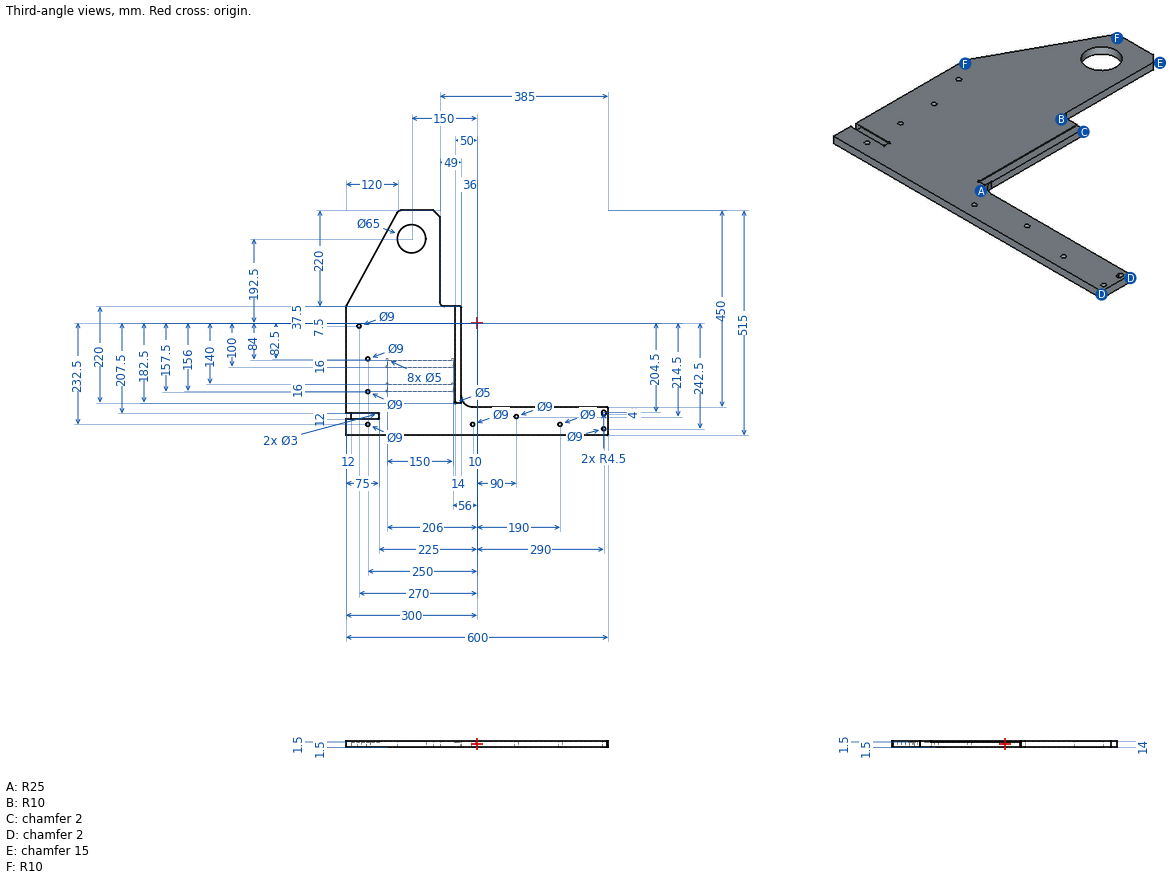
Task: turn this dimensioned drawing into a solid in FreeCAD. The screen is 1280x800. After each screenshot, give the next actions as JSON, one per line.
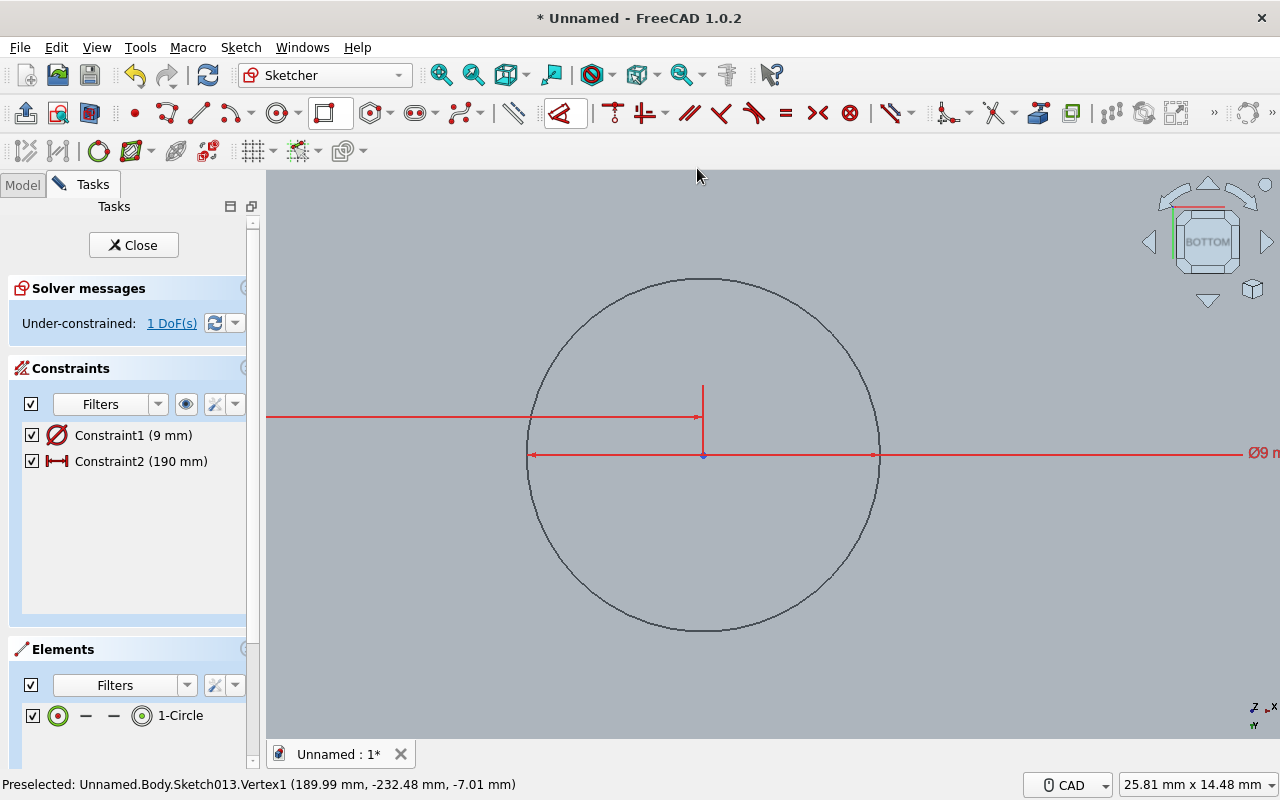
{"action": "left_click", "coordinate": [703, 455]}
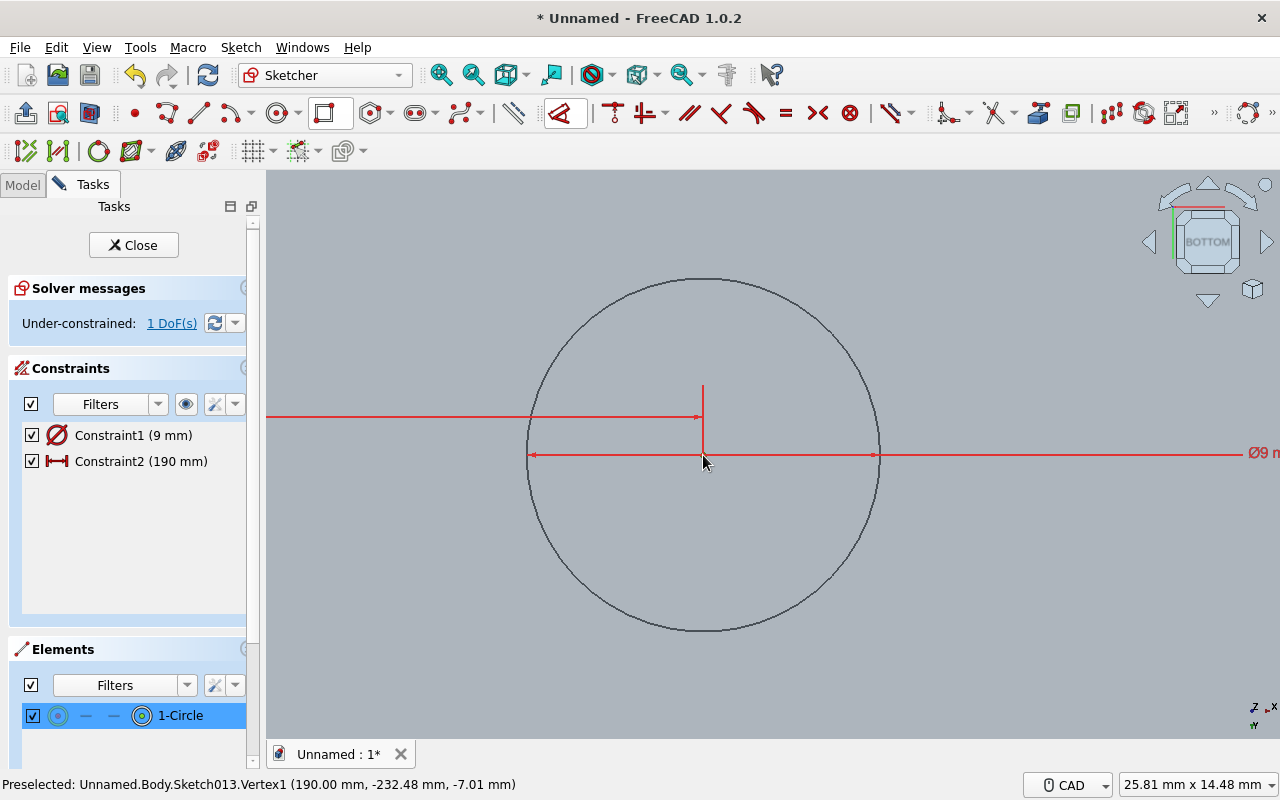
{"action": "left_click", "coordinate": [582, 114]}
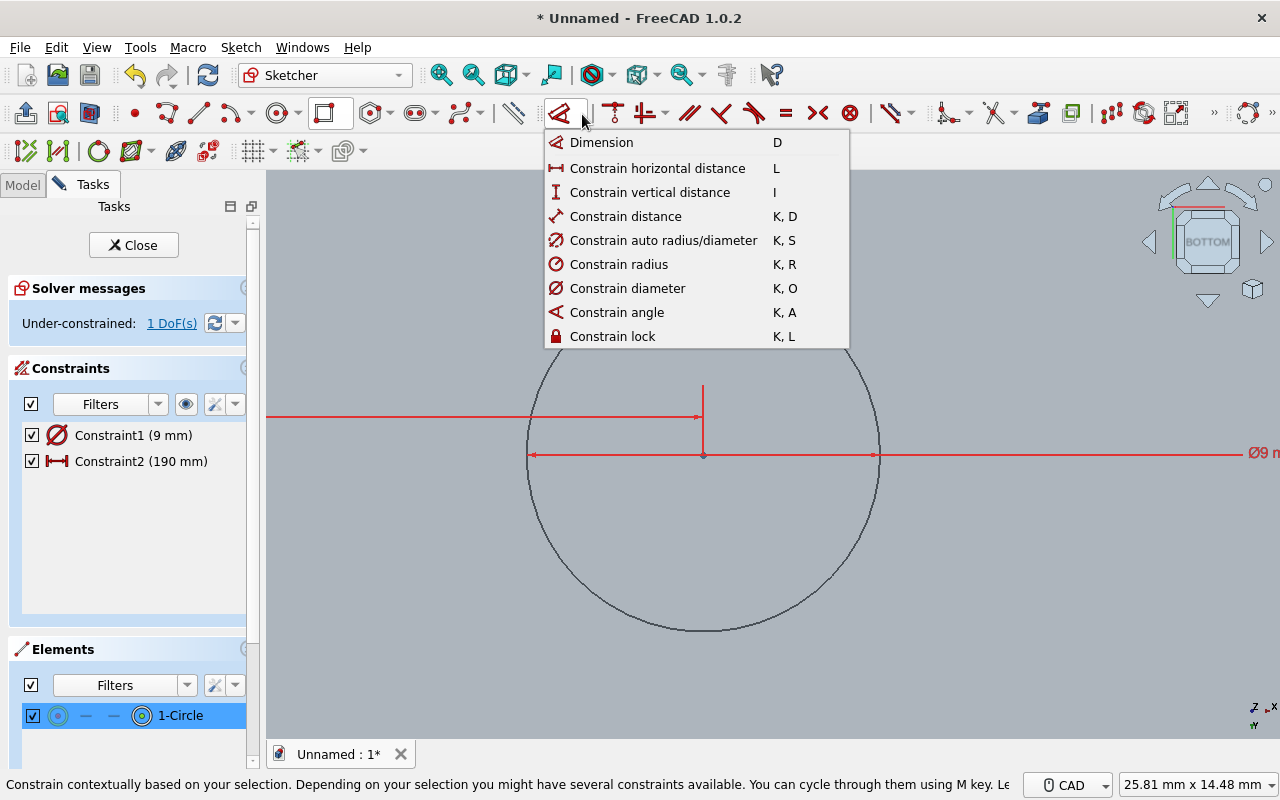
{"action": "left_click", "coordinate": [697, 192]}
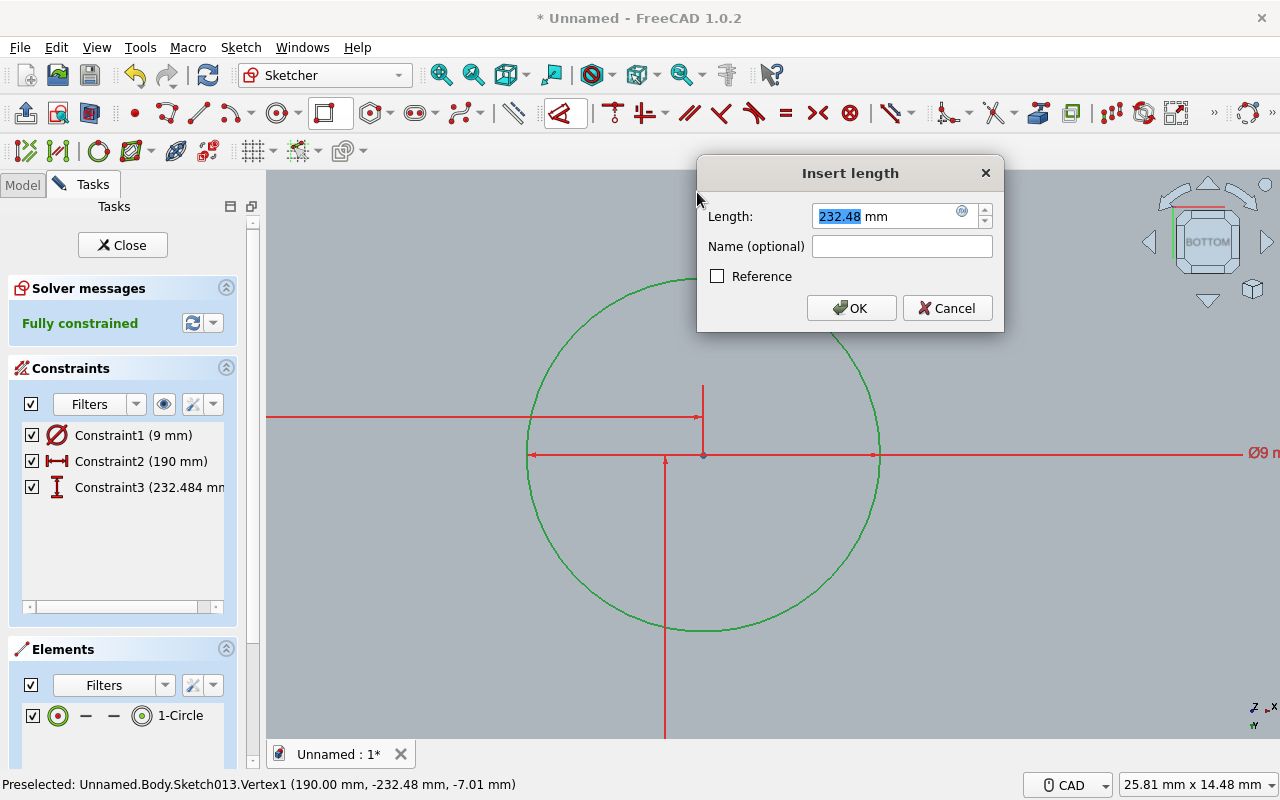
{"action": "type", "text": "232.5"}
{"action": "key", "text": "Return"}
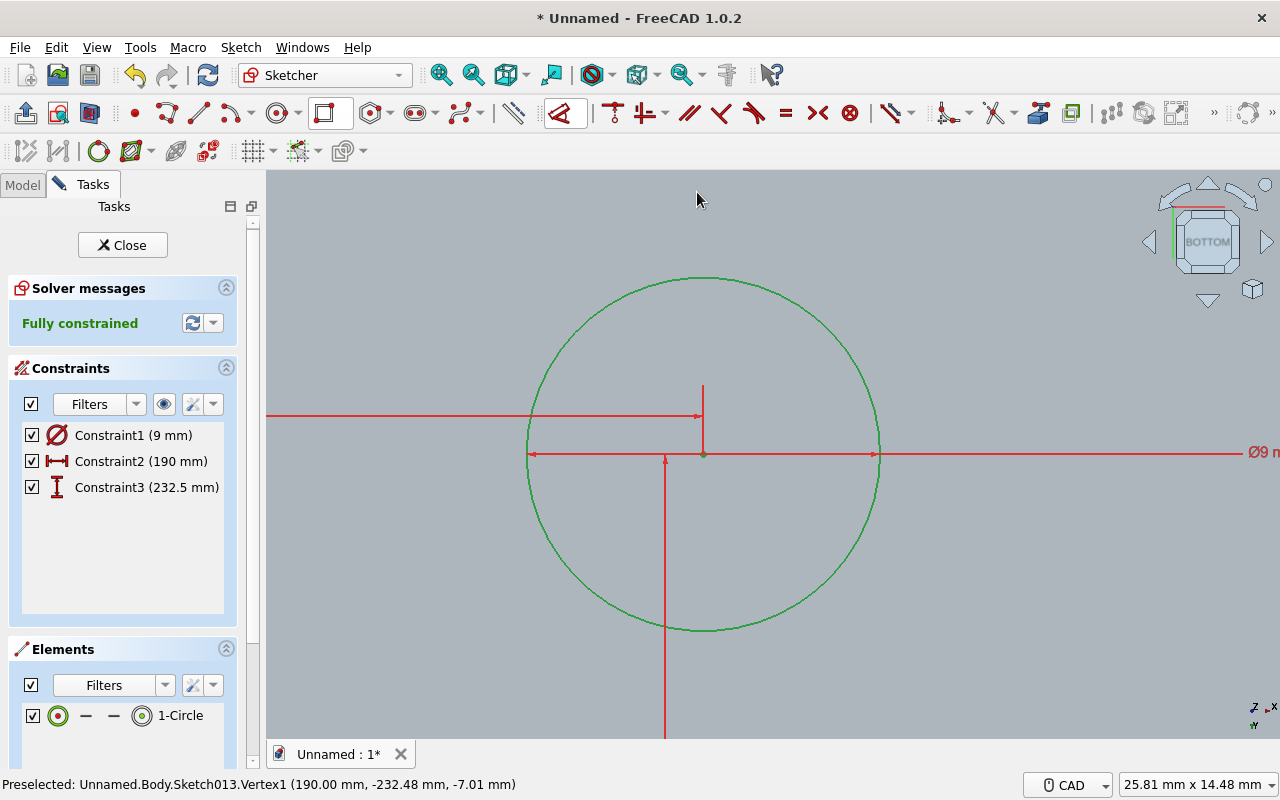
{"action": "left_click", "coordinate": [123, 245]}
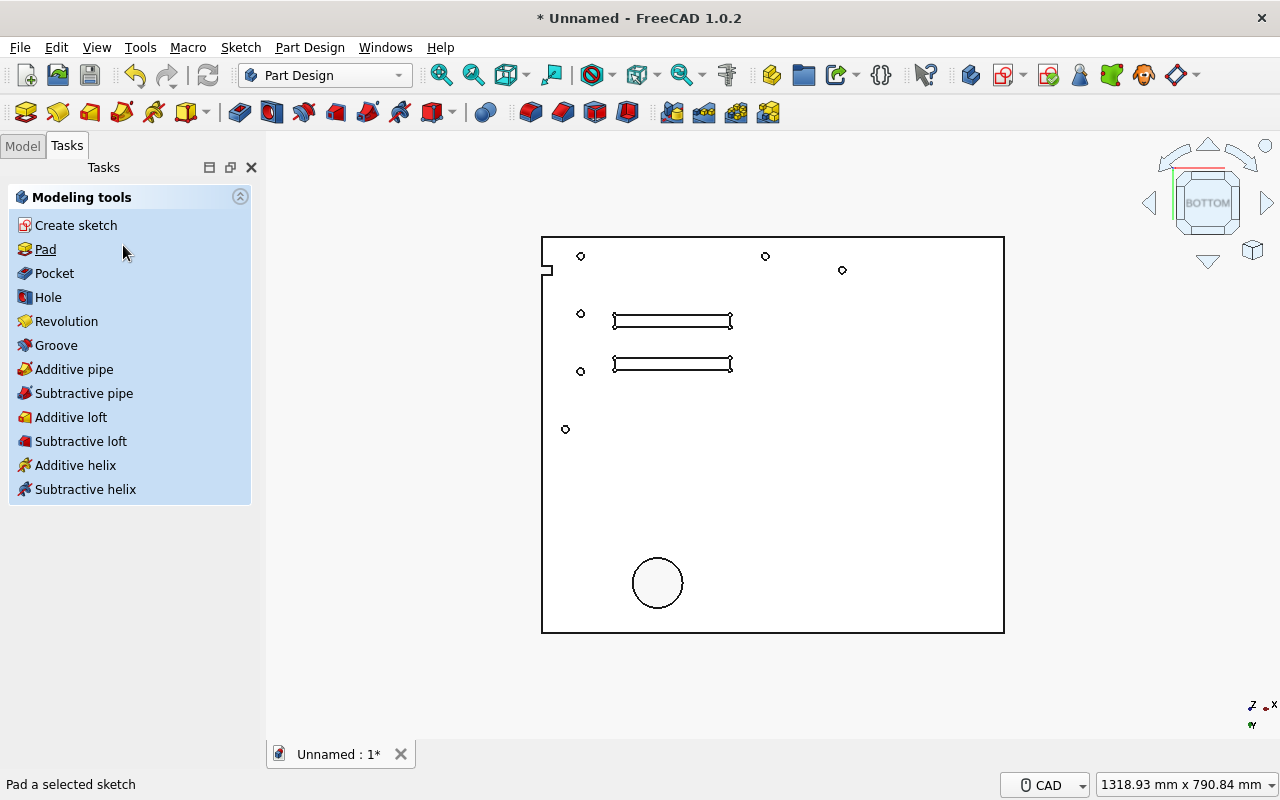
{"action": "left_click", "coordinate": [240, 112]}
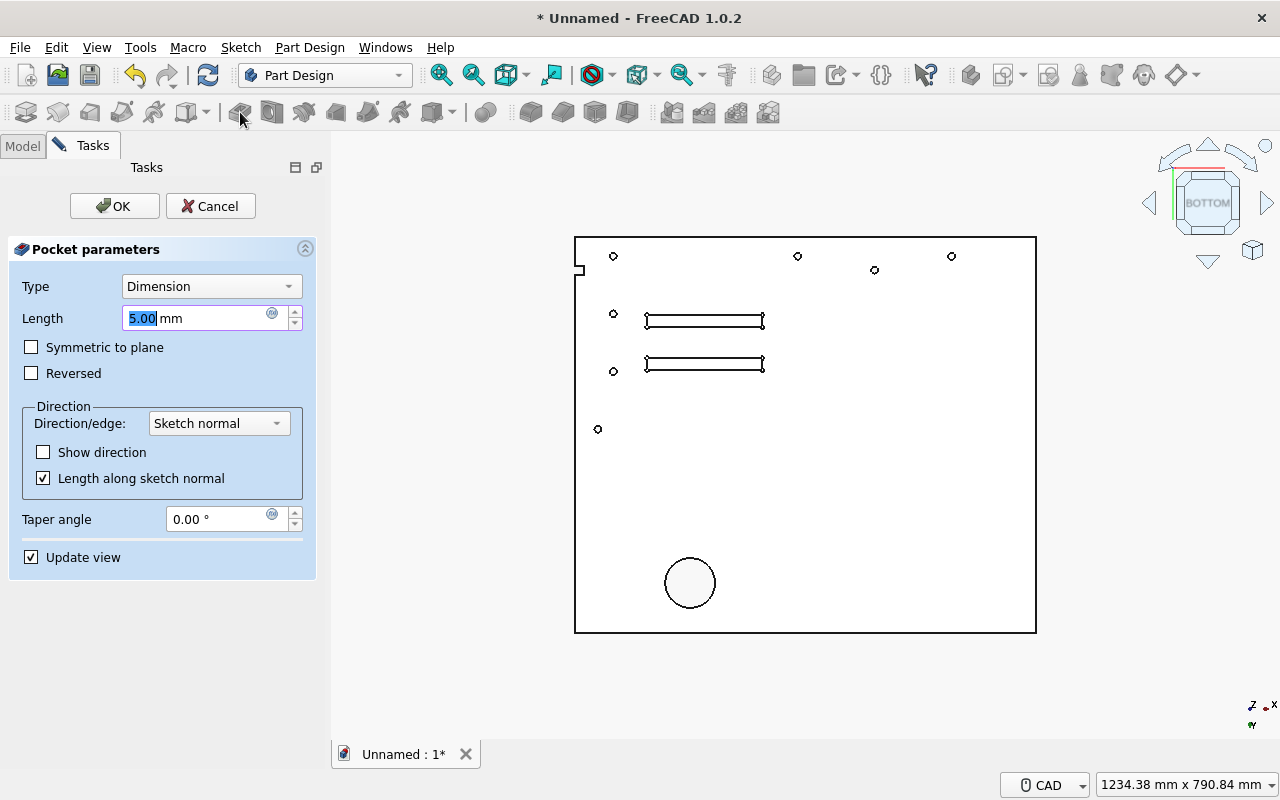
{"action": "left_click", "coordinate": [212, 286]}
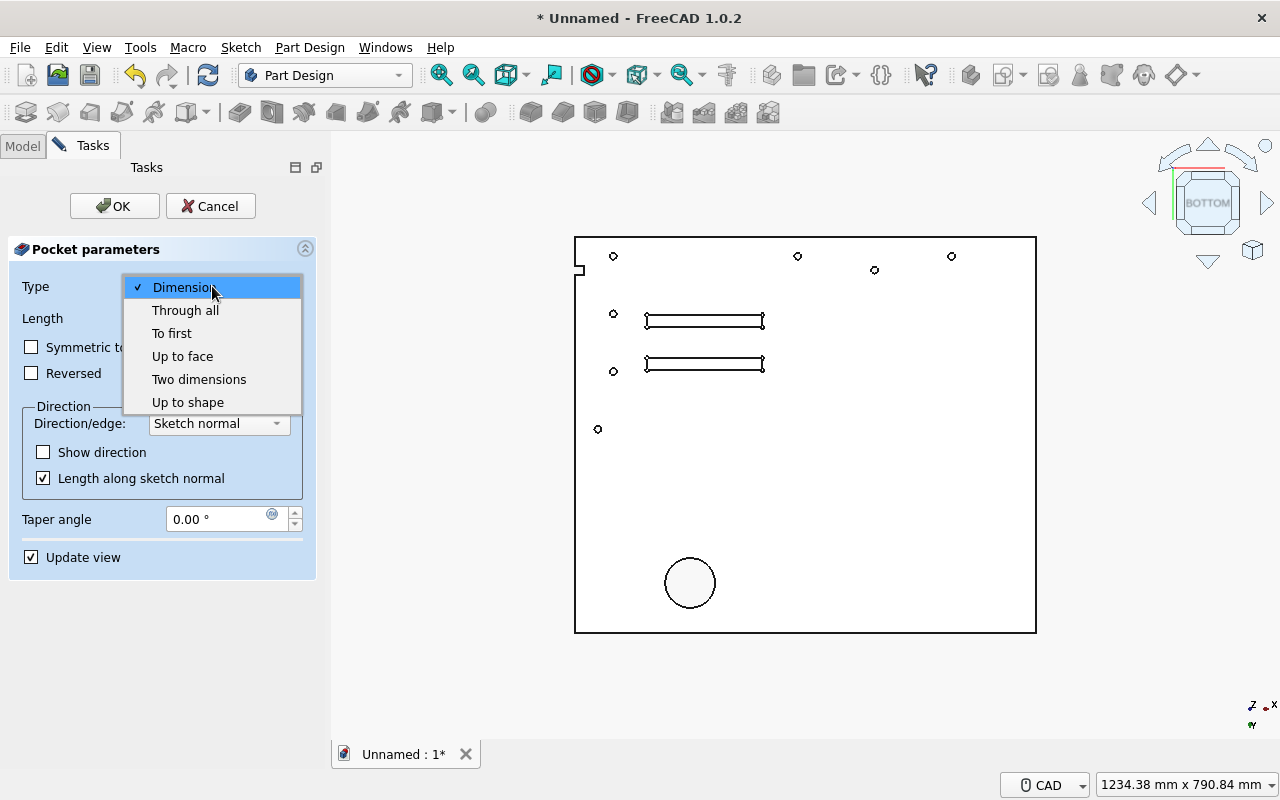
{"action": "left_click", "coordinate": [212, 334]}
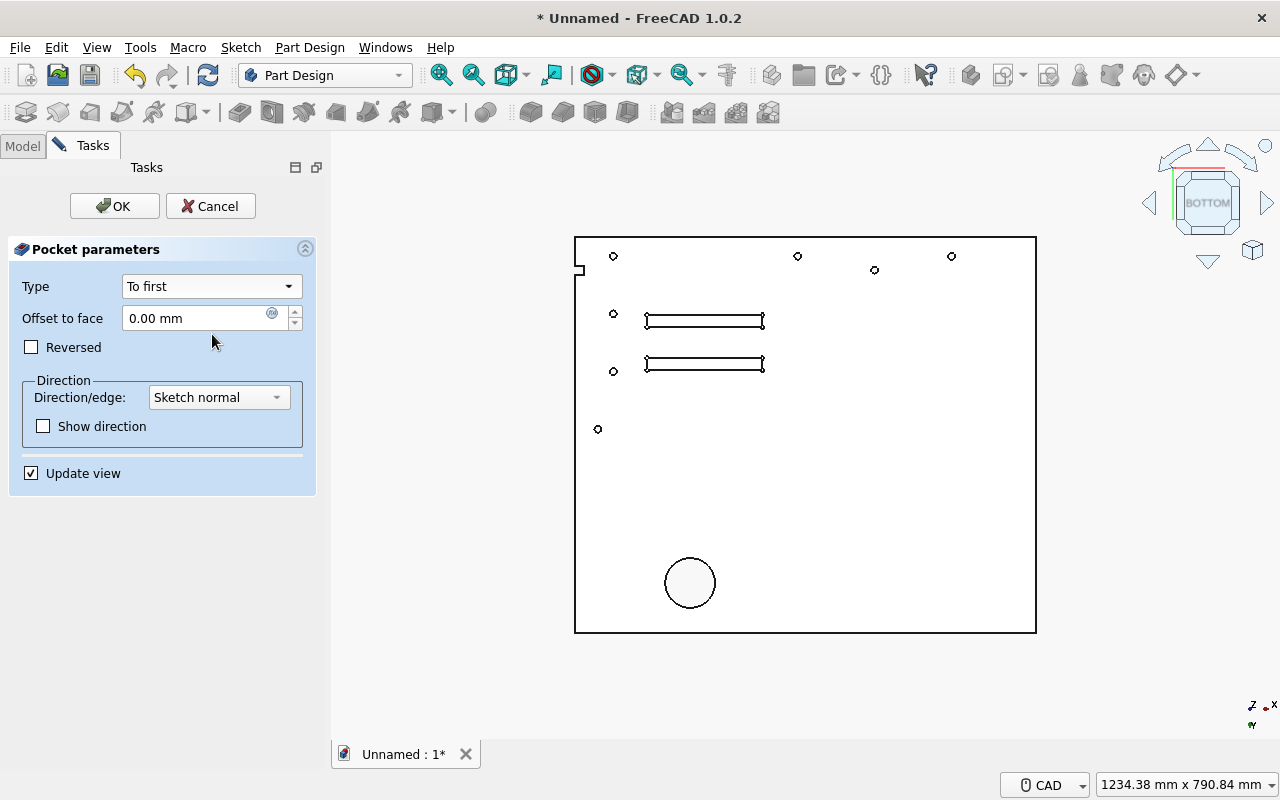
{"action": "left_click", "coordinate": [115, 206]}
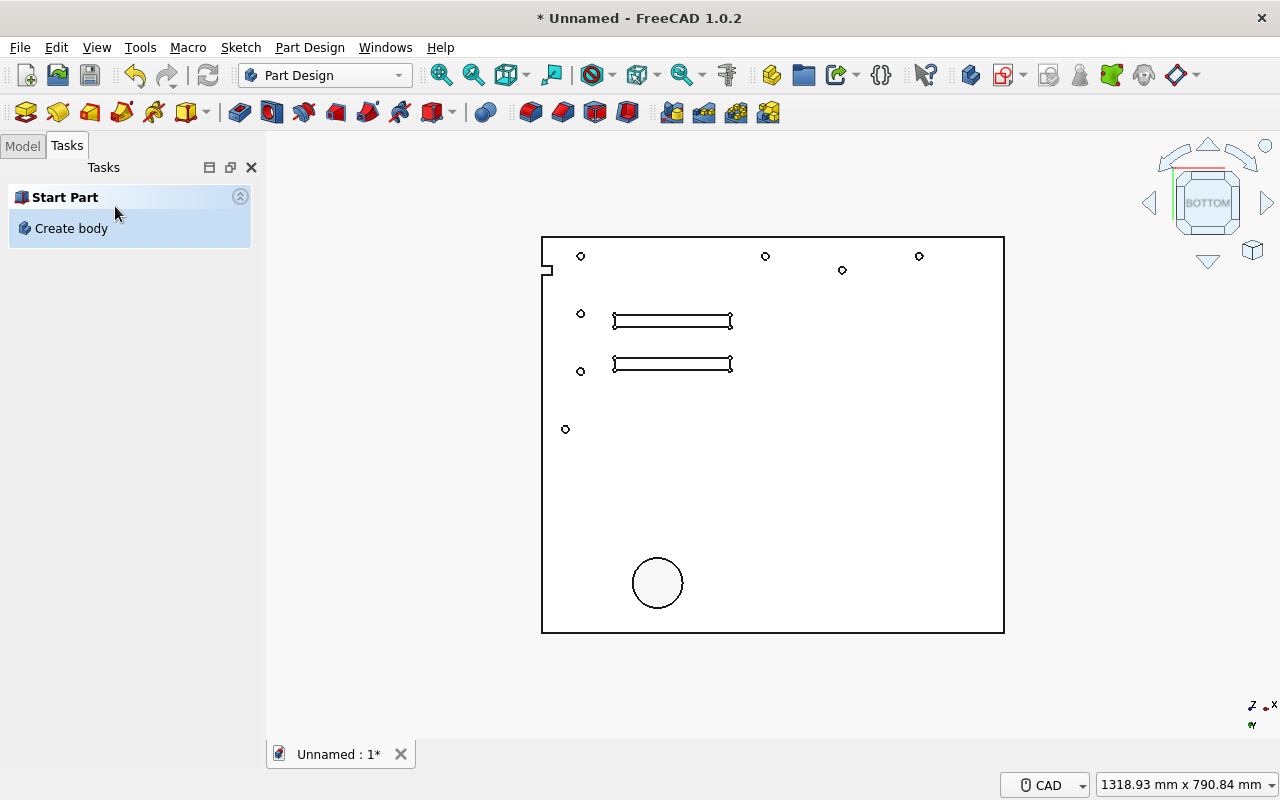
{"action": "left_click", "coordinate": [839, 491]}